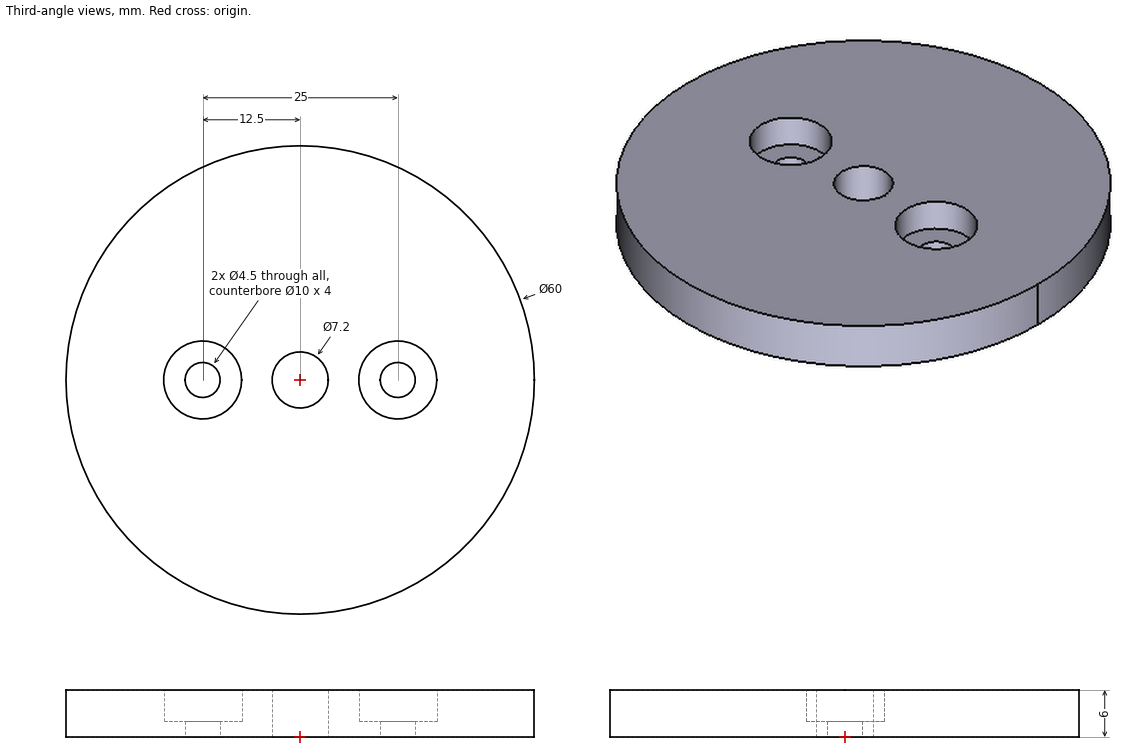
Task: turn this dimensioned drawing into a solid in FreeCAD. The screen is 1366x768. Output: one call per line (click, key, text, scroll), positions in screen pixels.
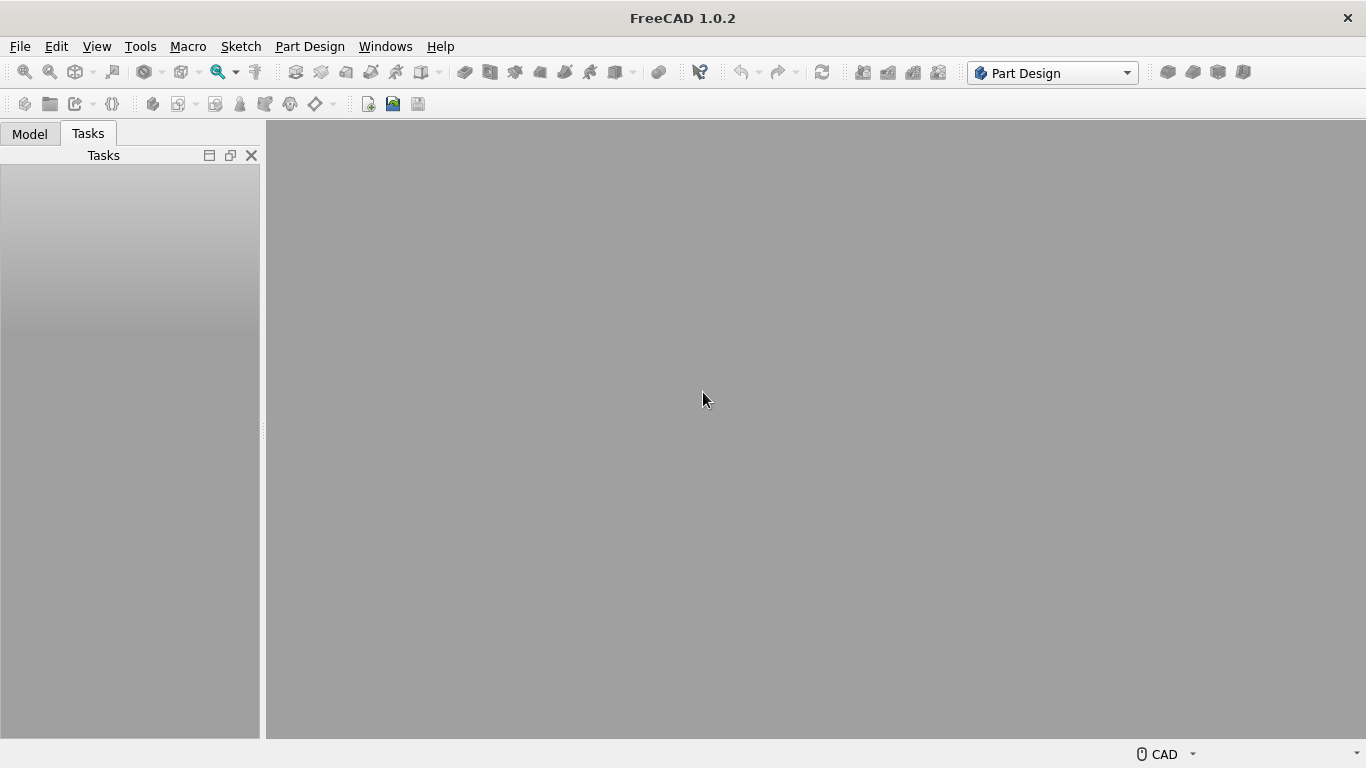
click(368, 104)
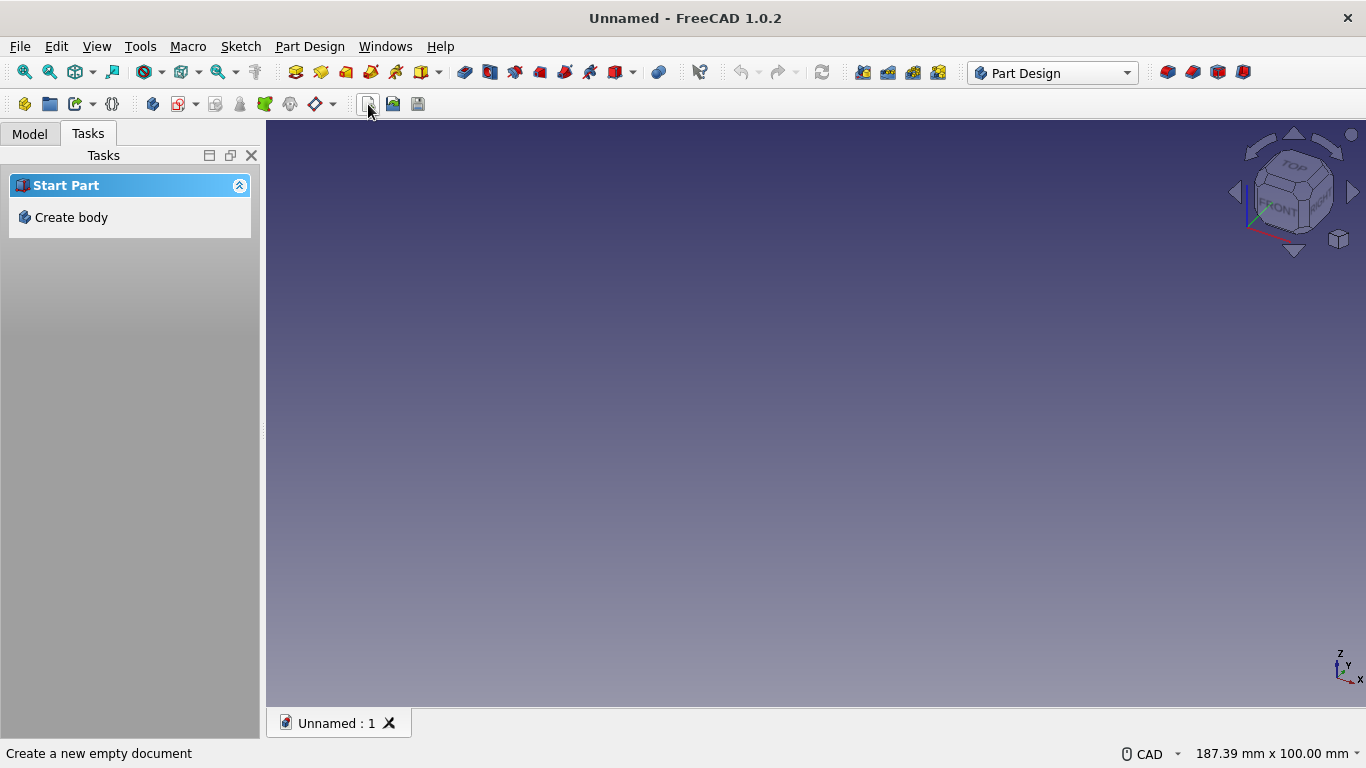
click(178, 104)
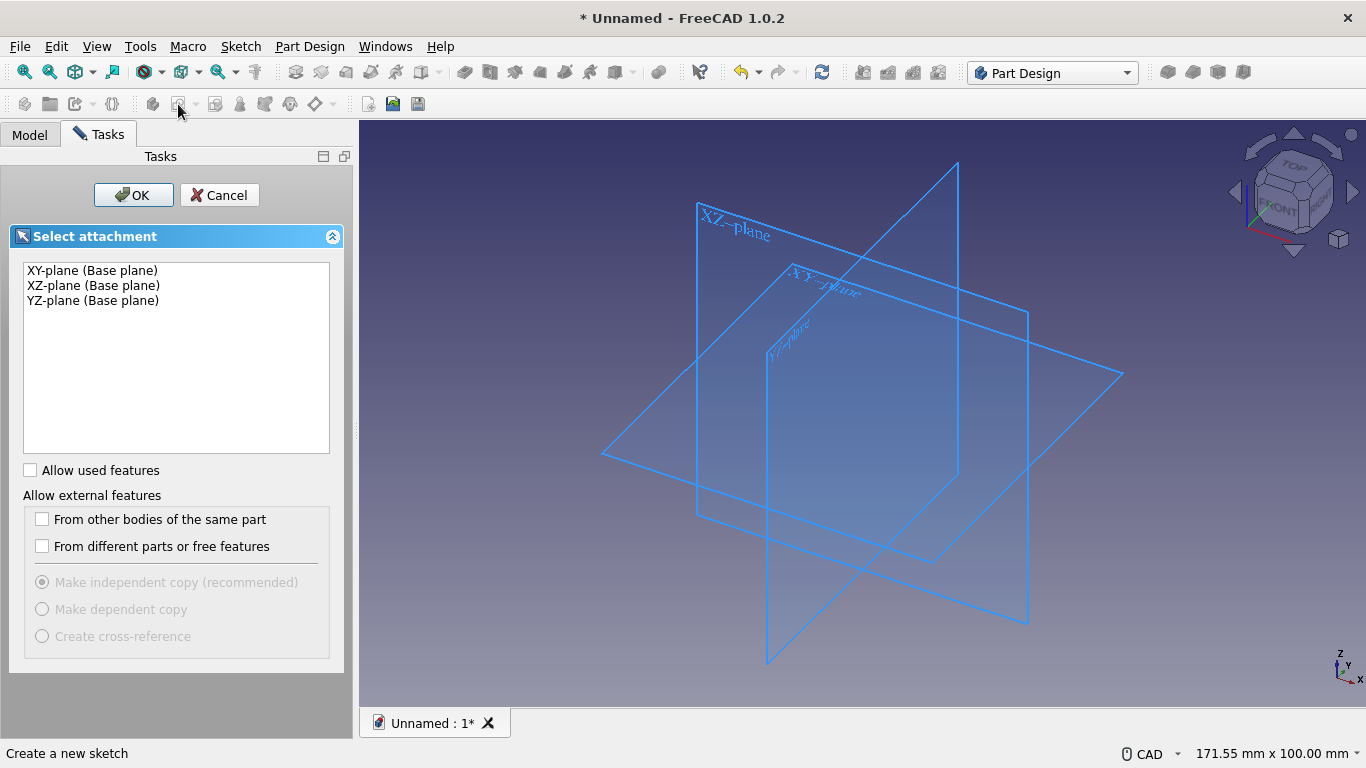
click(84, 270)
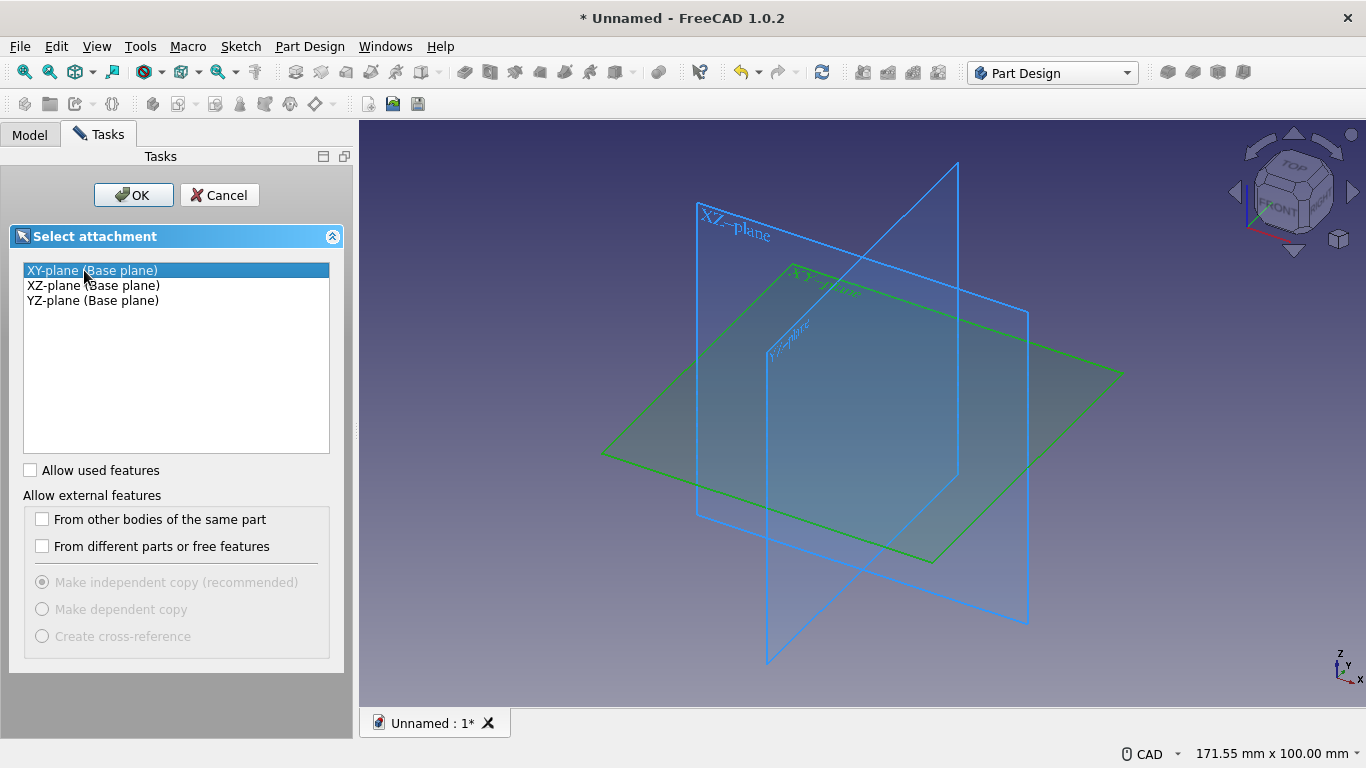
click(134, 195)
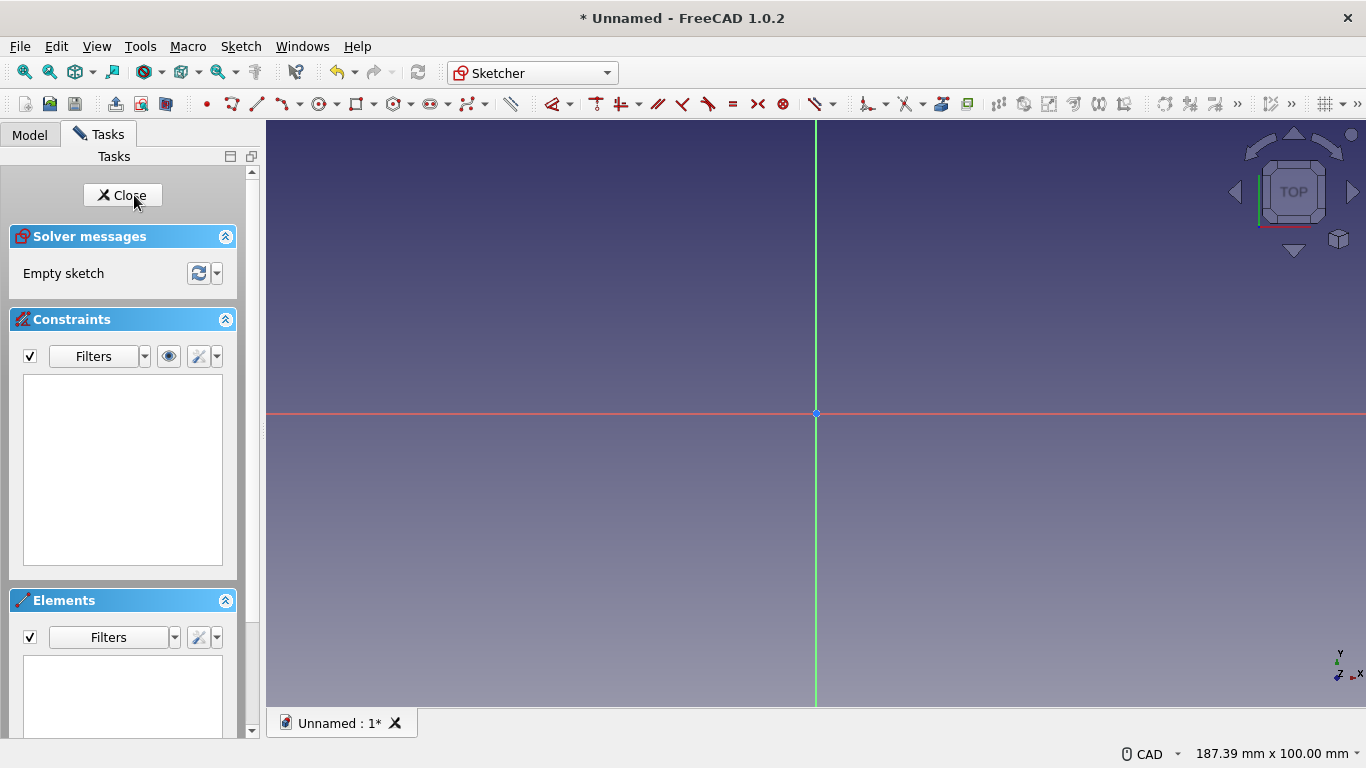
click(318, 104)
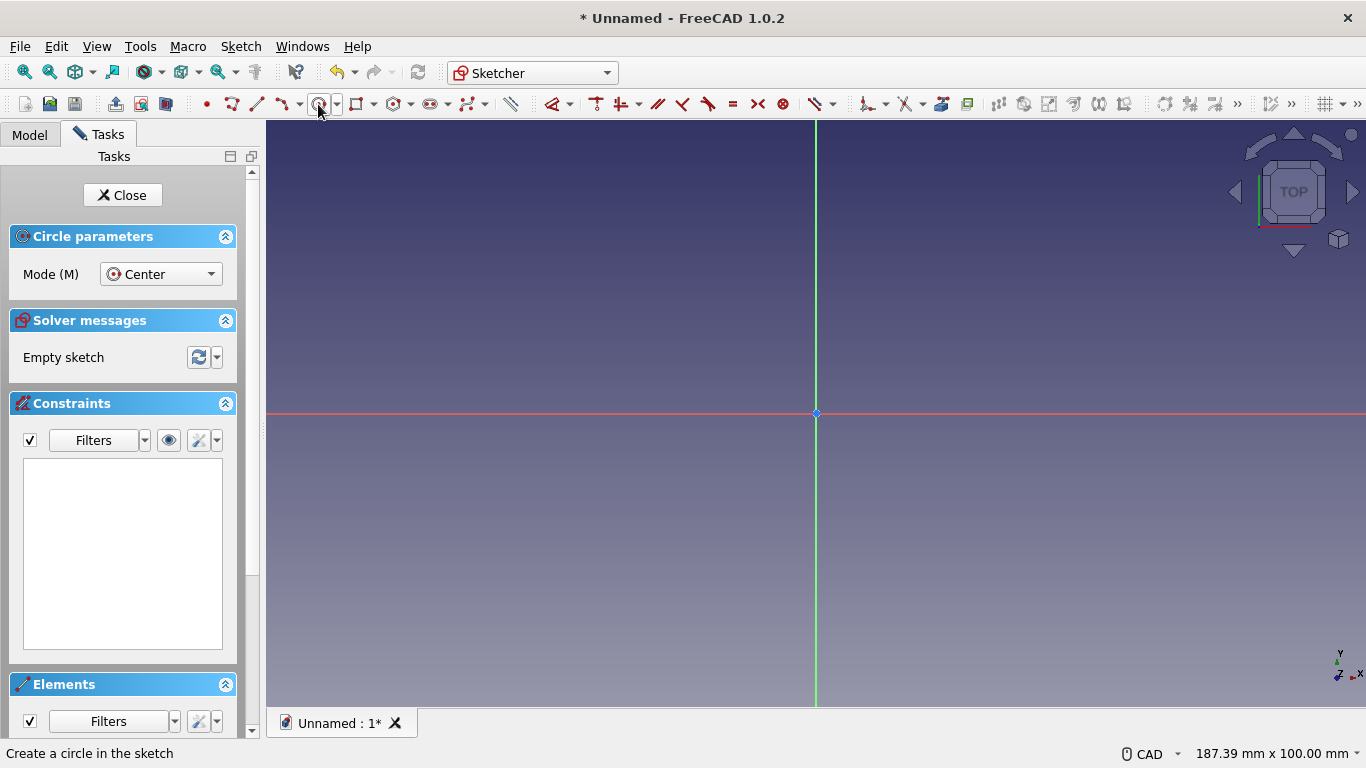
click(816, 414)
click(941, 289)
key(Escape)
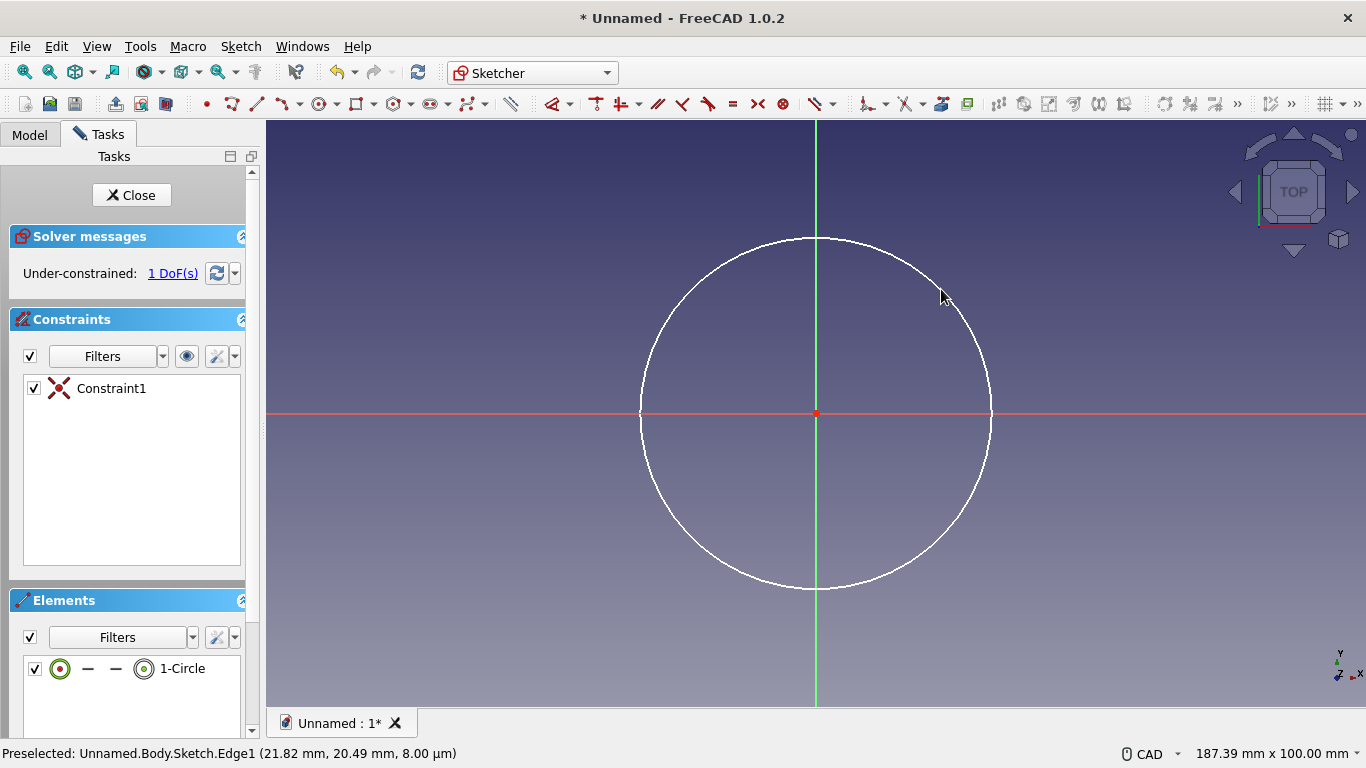
click(552, 104)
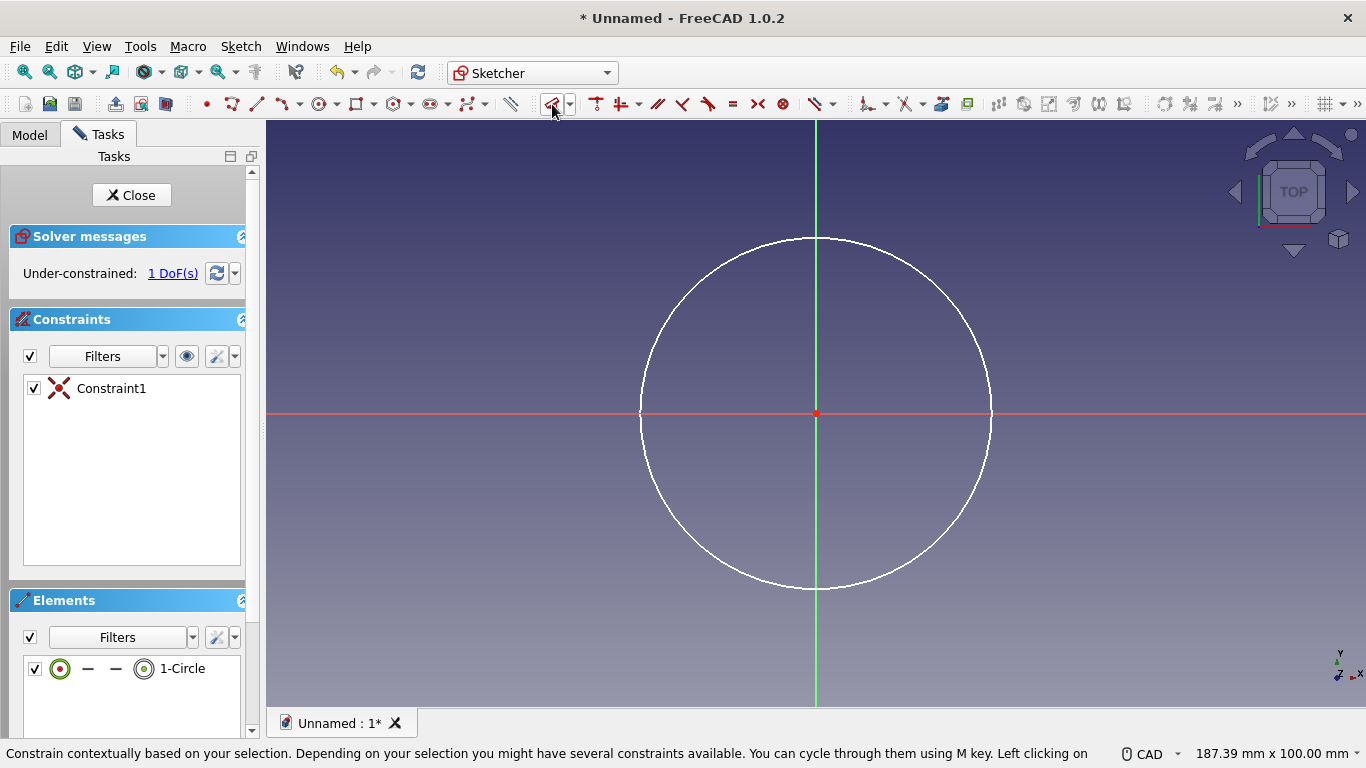
click(940, 289)
click(963, 266)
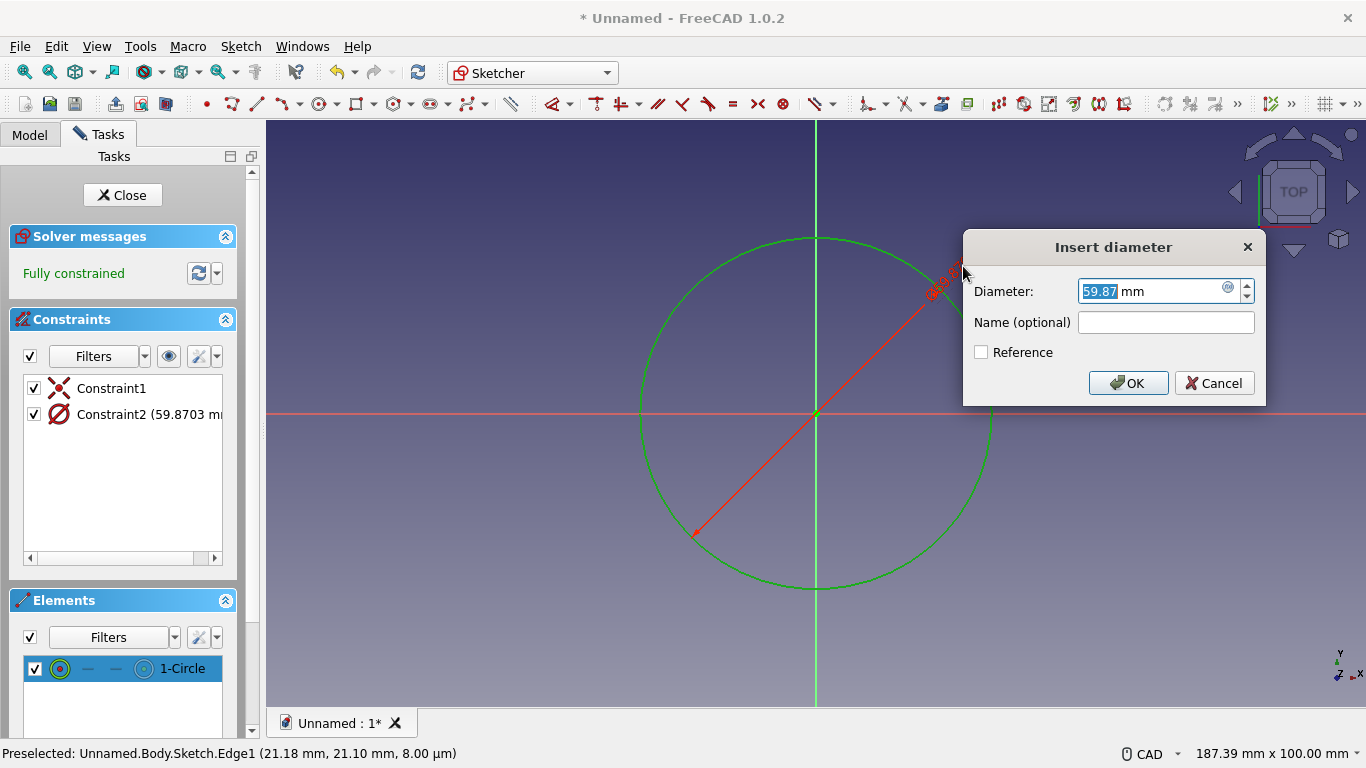
text(60)
key(Return)
key(Escape)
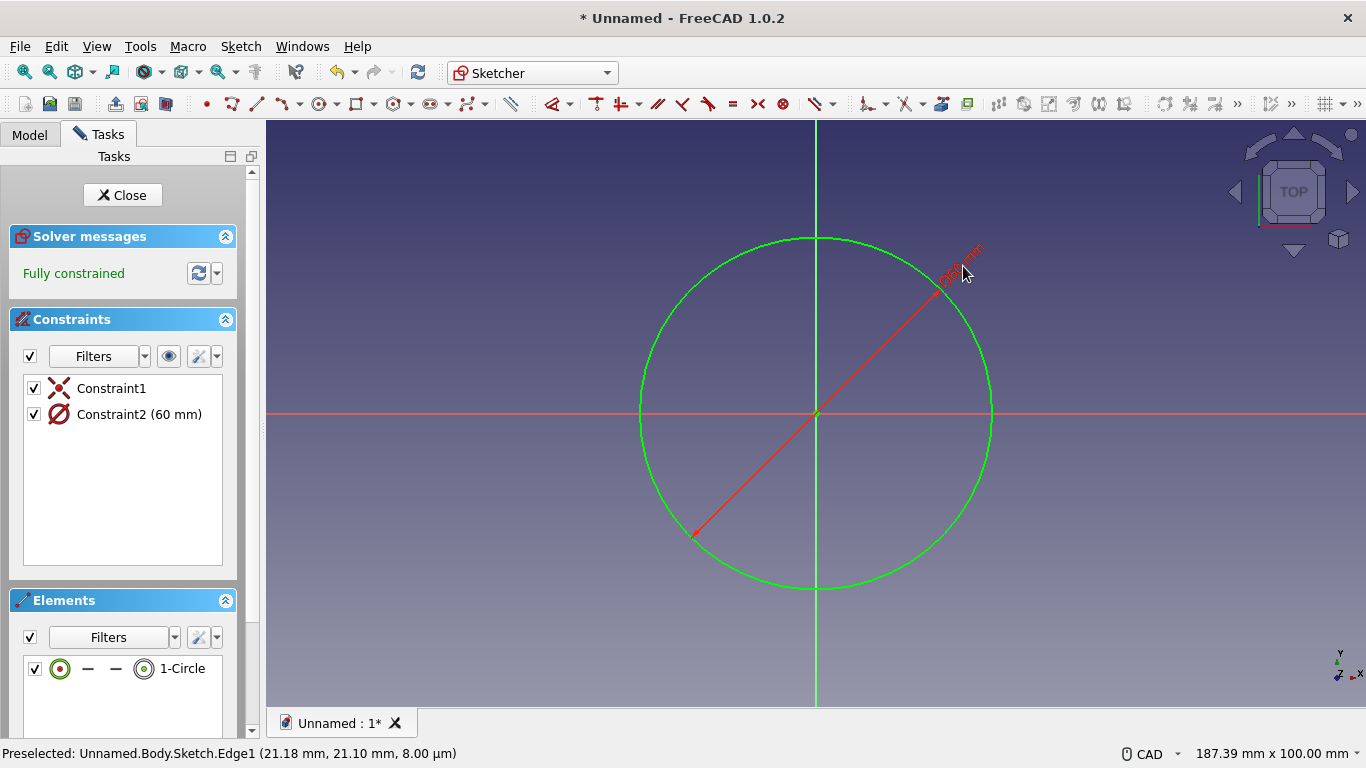
click(123, 195)